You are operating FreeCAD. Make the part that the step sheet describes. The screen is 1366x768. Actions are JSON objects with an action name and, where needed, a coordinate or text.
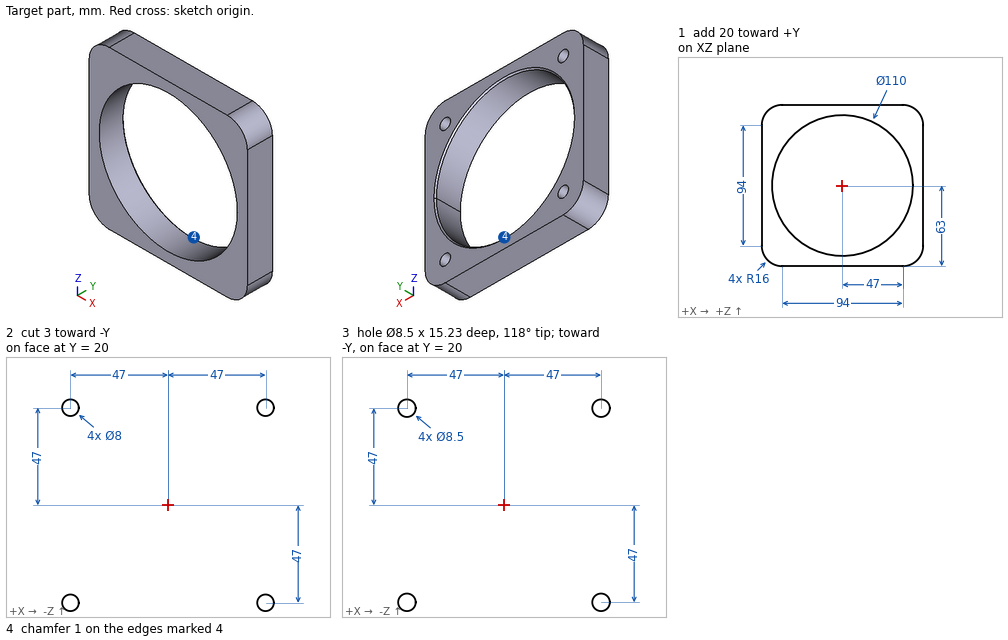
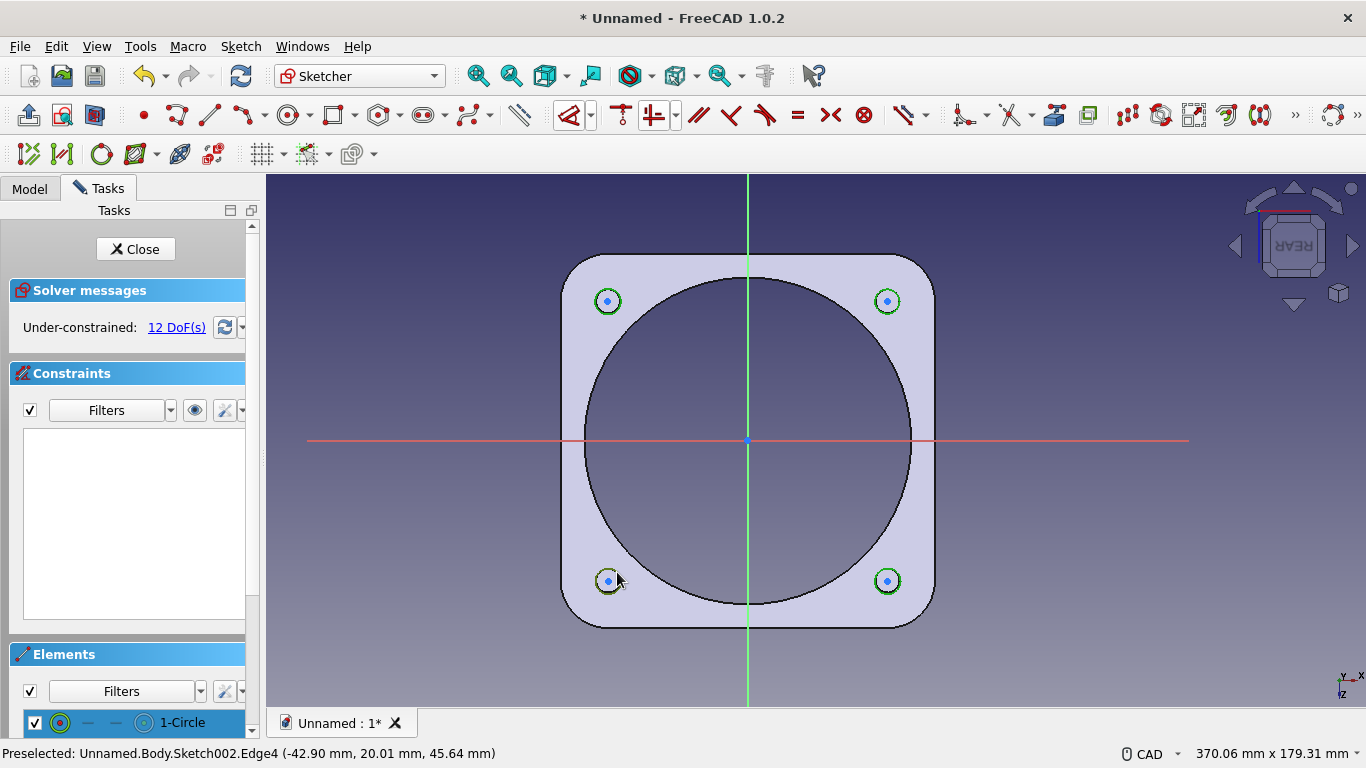
{"action": "left_click", "coordinate": [798, 116]}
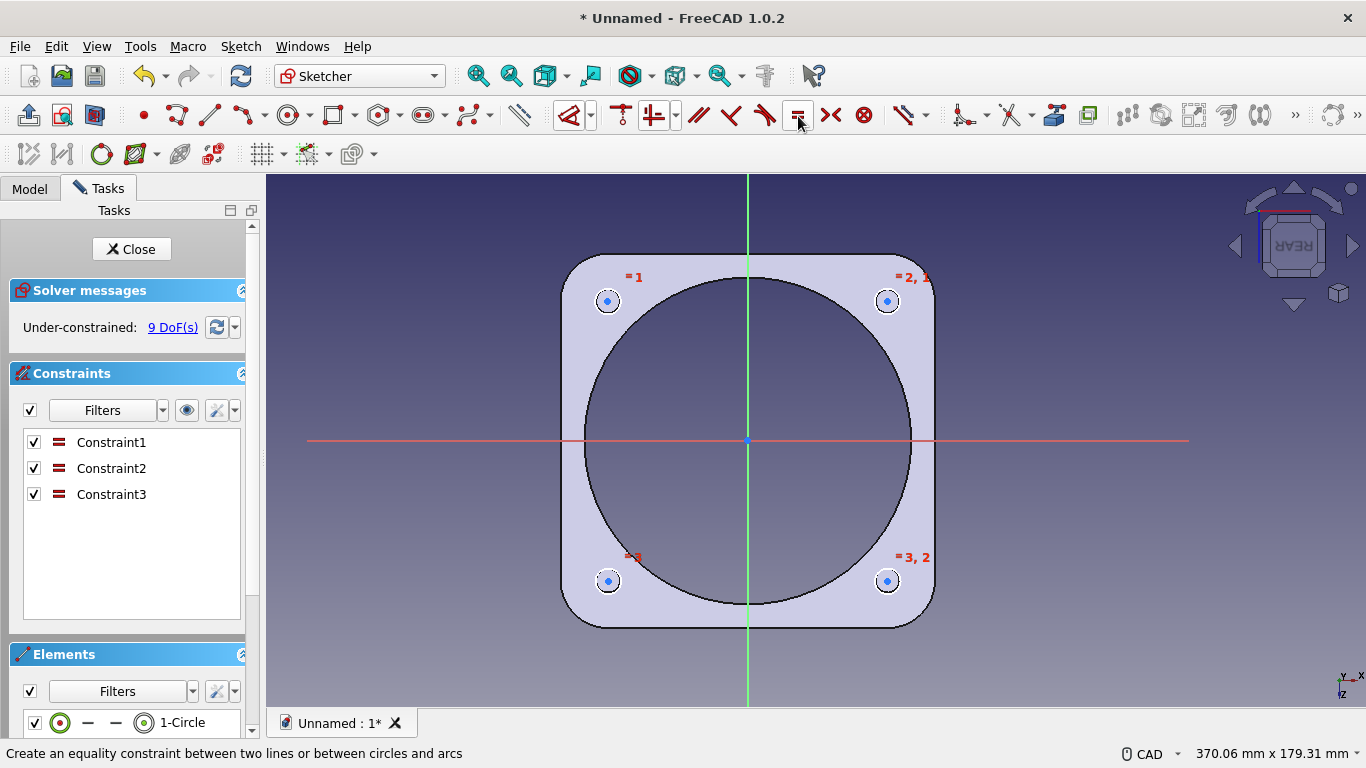
{"action": "left_click", "coordinate": [608, 302]}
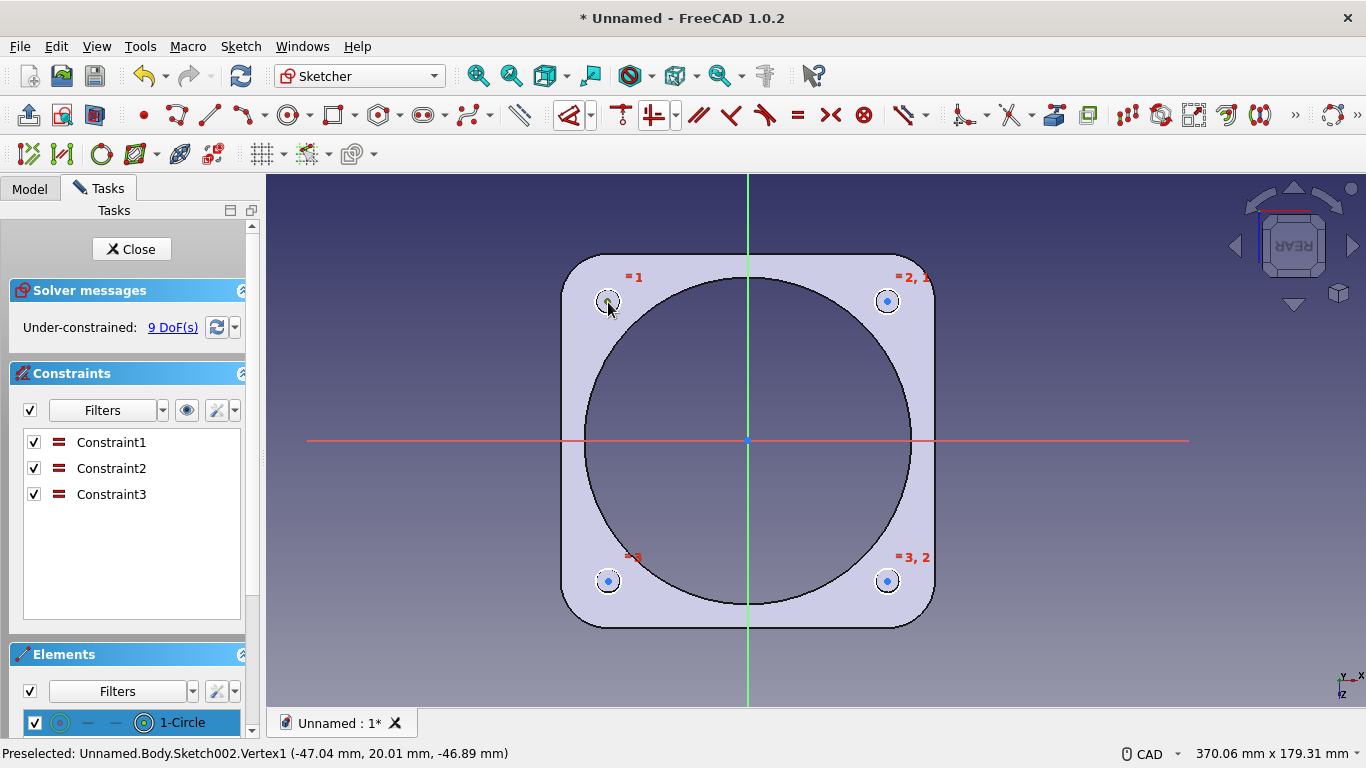
{"action": "left_click", "coordinate": [887, 302]}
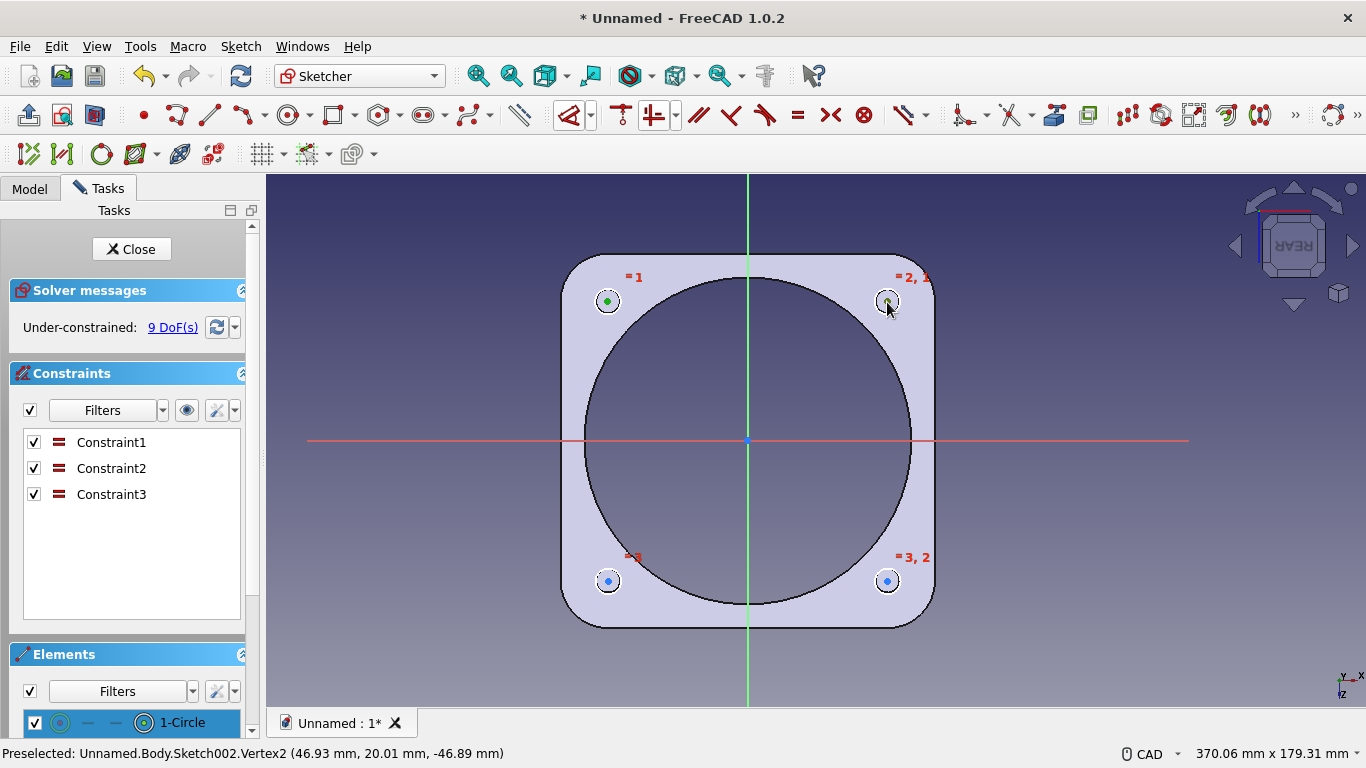
{"action": "key", "text": "h"}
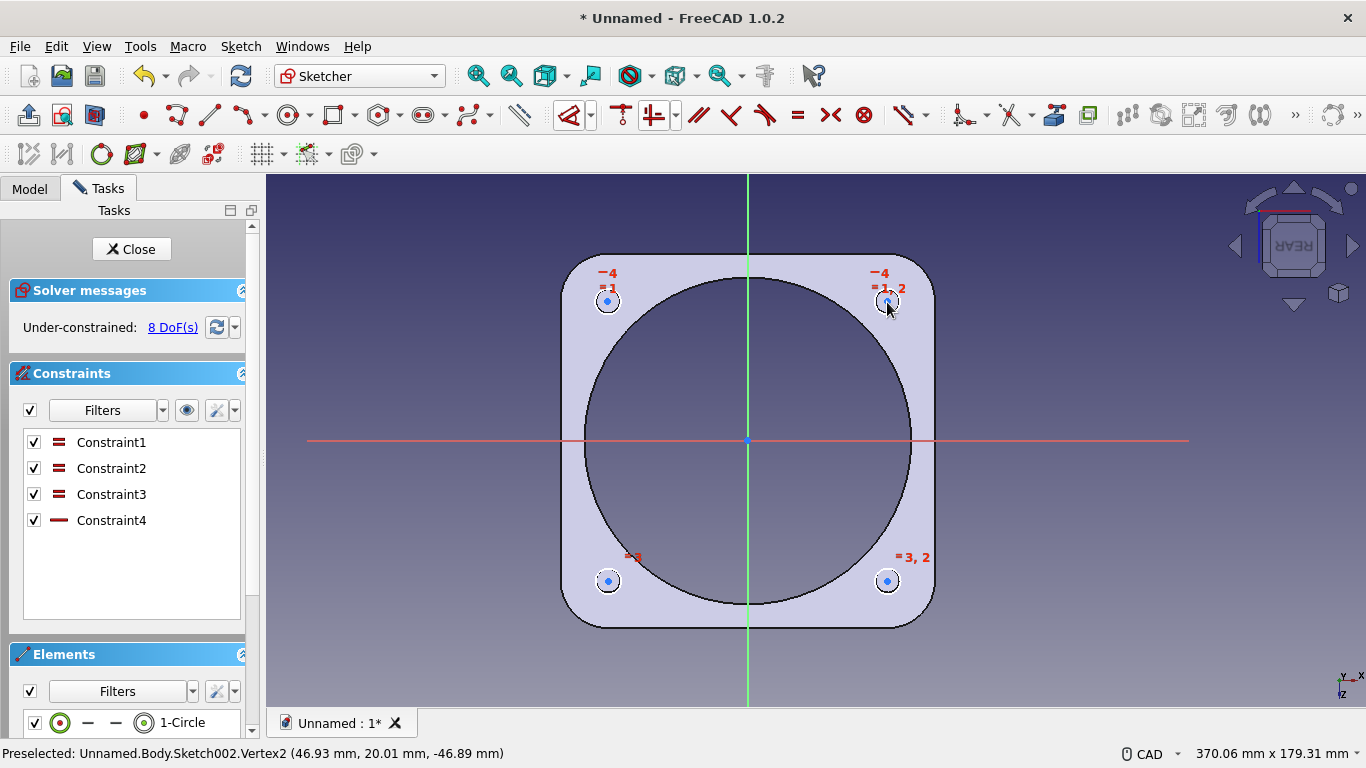
{"action": "left_click", "coordinate": [887, 302]}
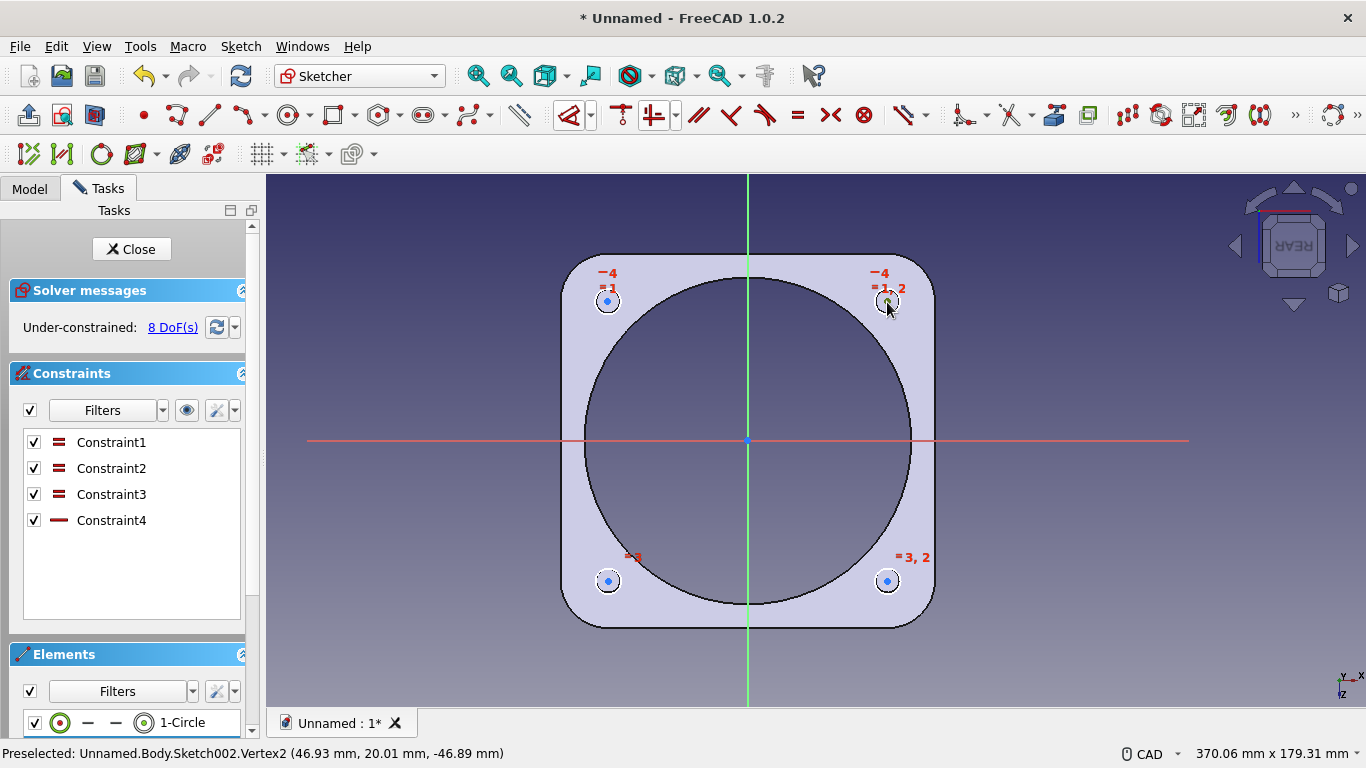
{"action": "left_click", "coordinate": [888, 581]}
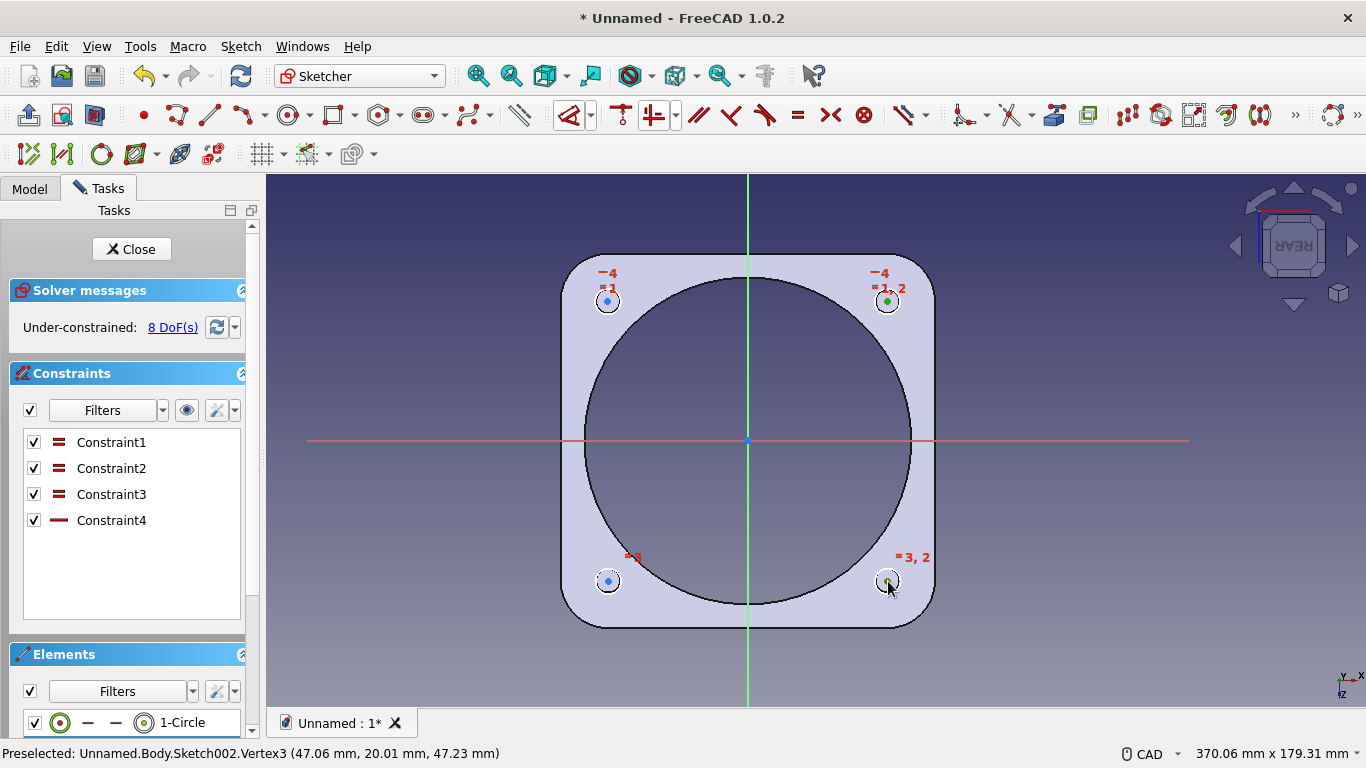
{"action": "left_click", "coordinate": [676, 116]}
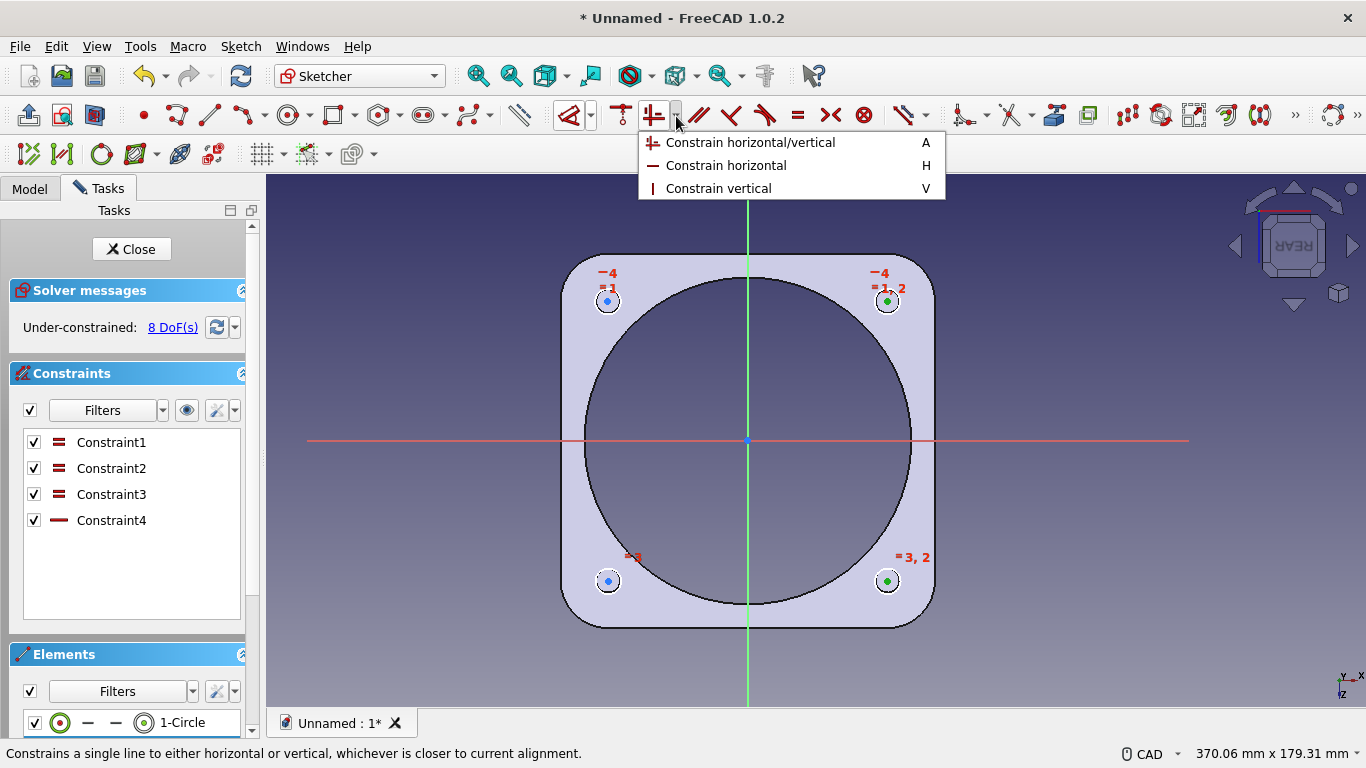
{"action": "left_click", "coordinate": [792, 188]}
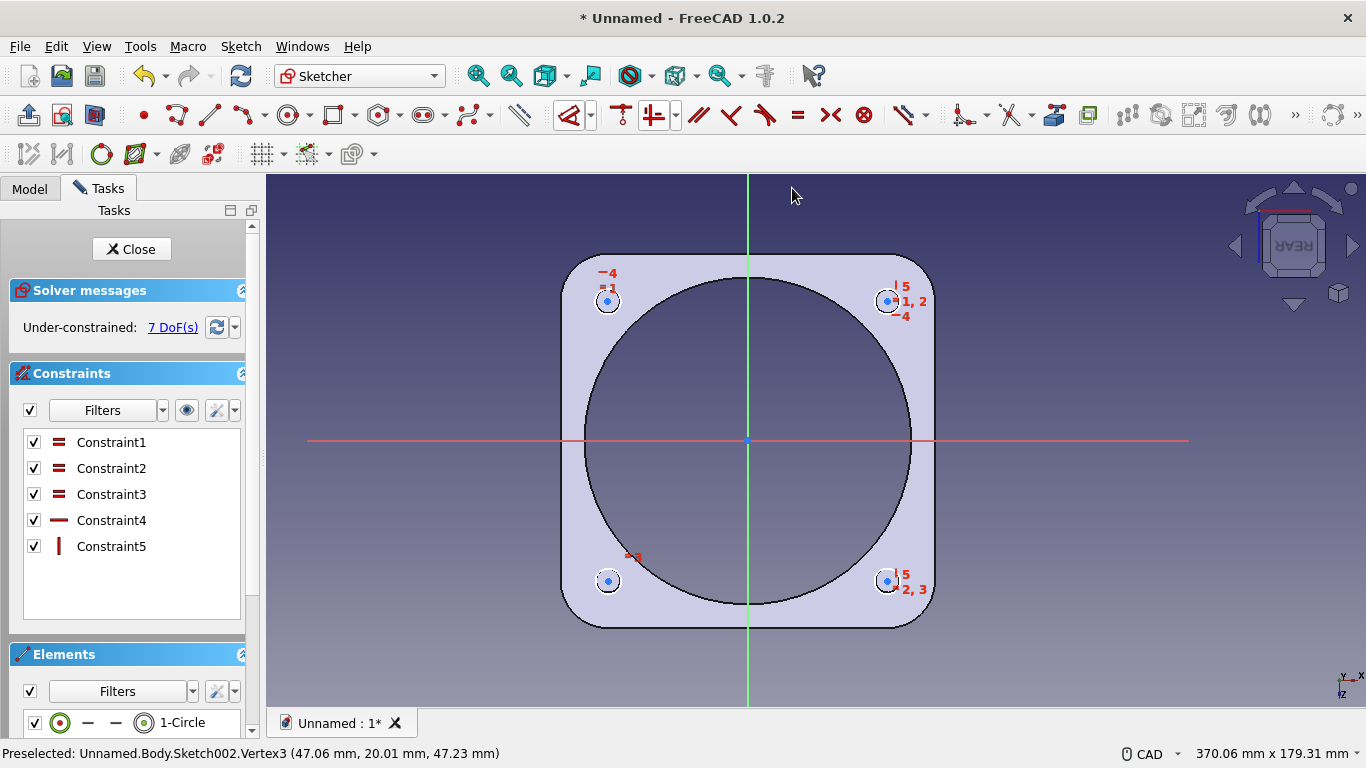
{"action": "left_click", "coordinate": [608, 302]}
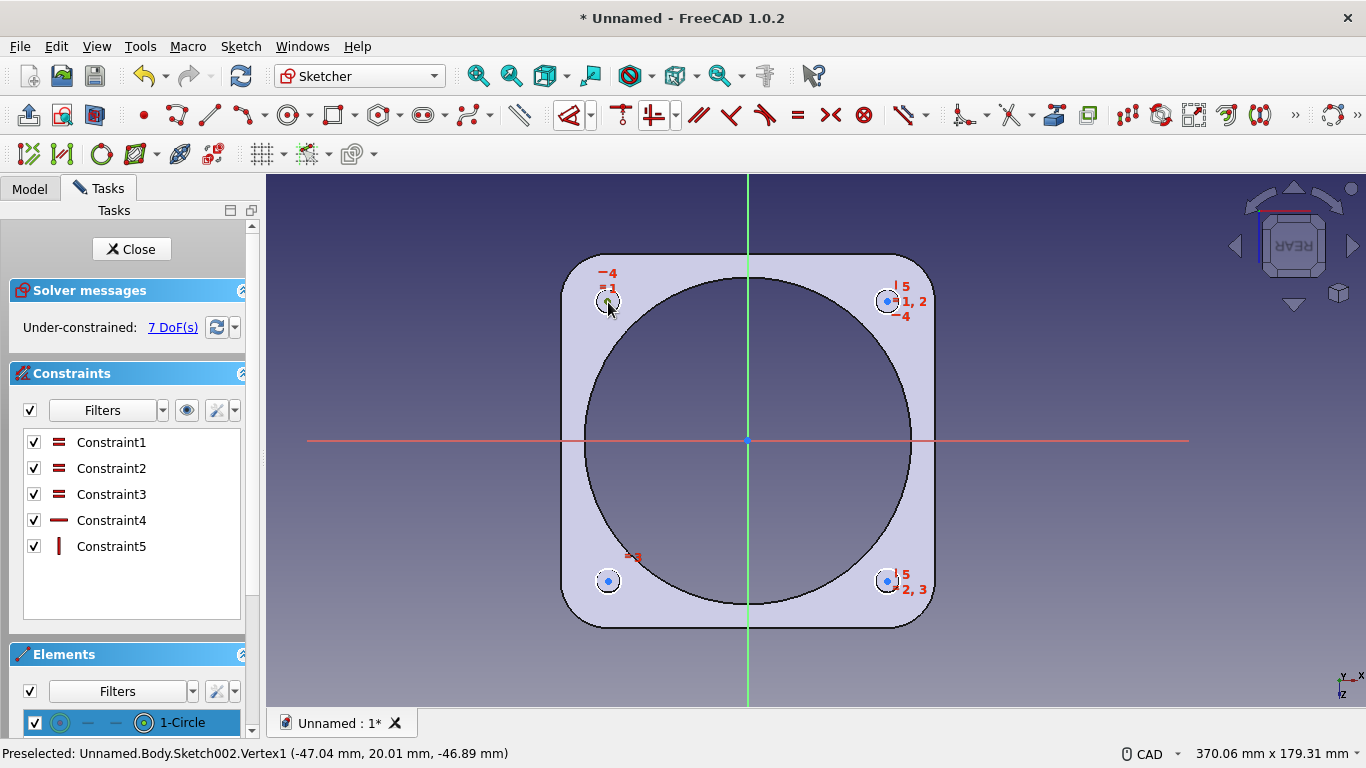
{"action": "left_click", "coordinate": [608, 581]}